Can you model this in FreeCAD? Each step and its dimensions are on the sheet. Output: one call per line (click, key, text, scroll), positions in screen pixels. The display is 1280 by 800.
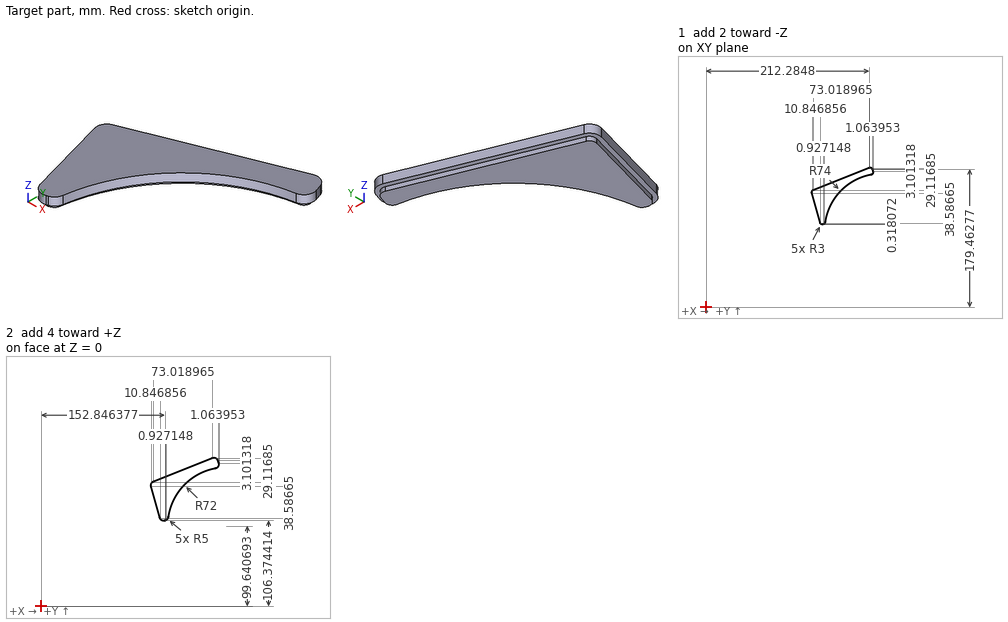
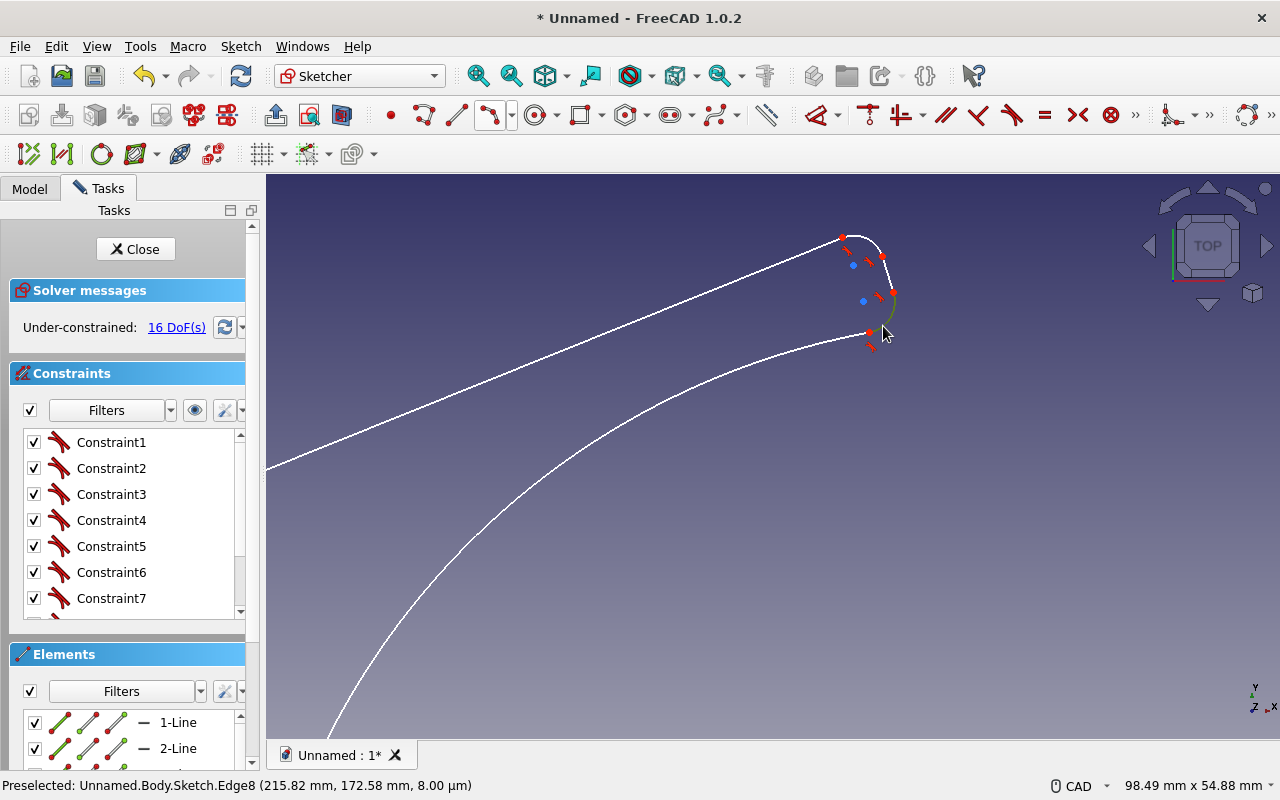
click(875, 244)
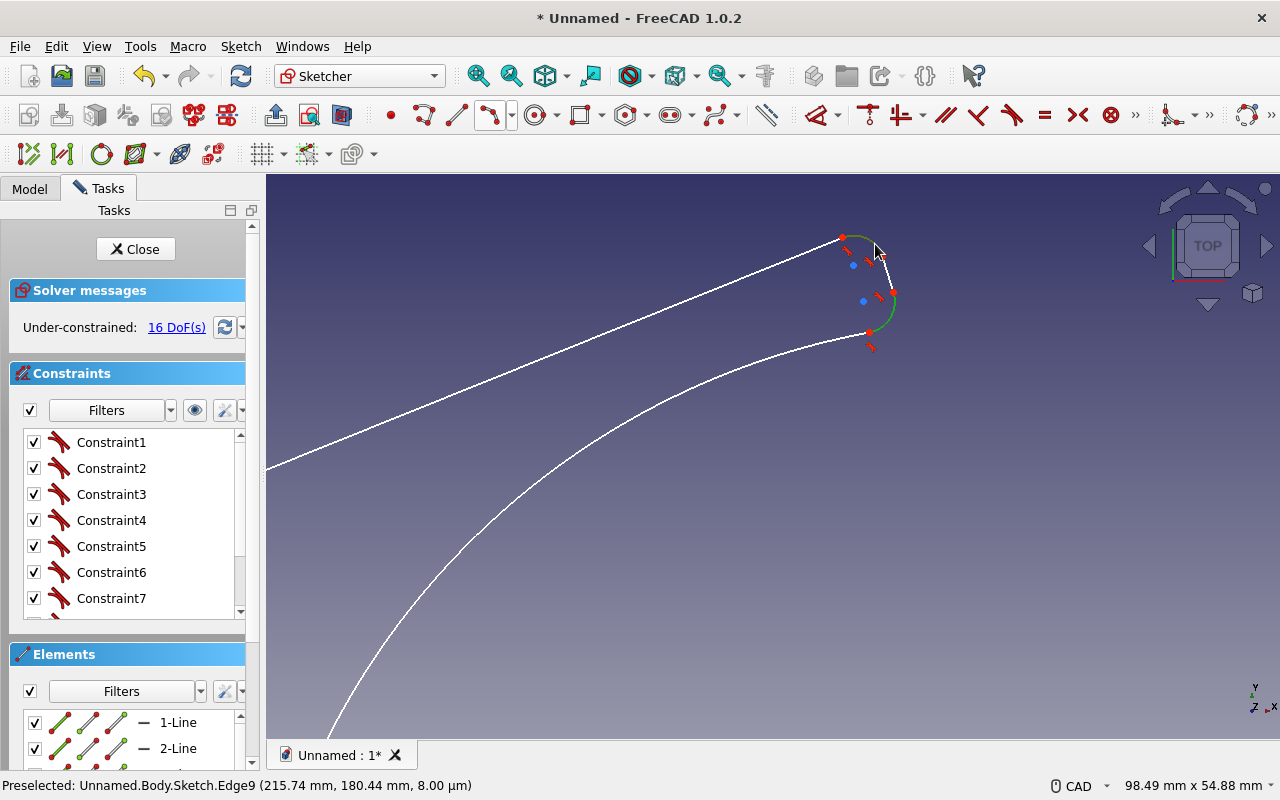
scroll(885, 326, down, 4)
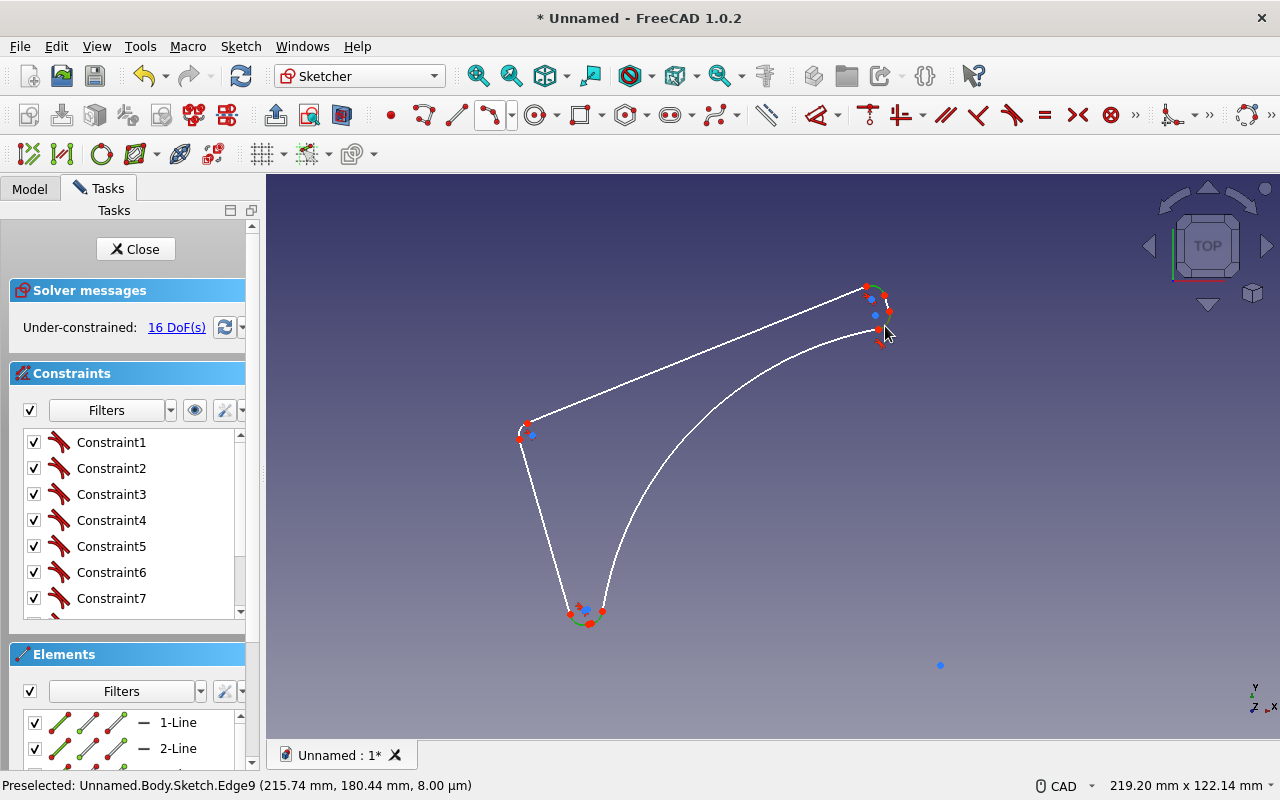
scroll(522, 426, up, 5)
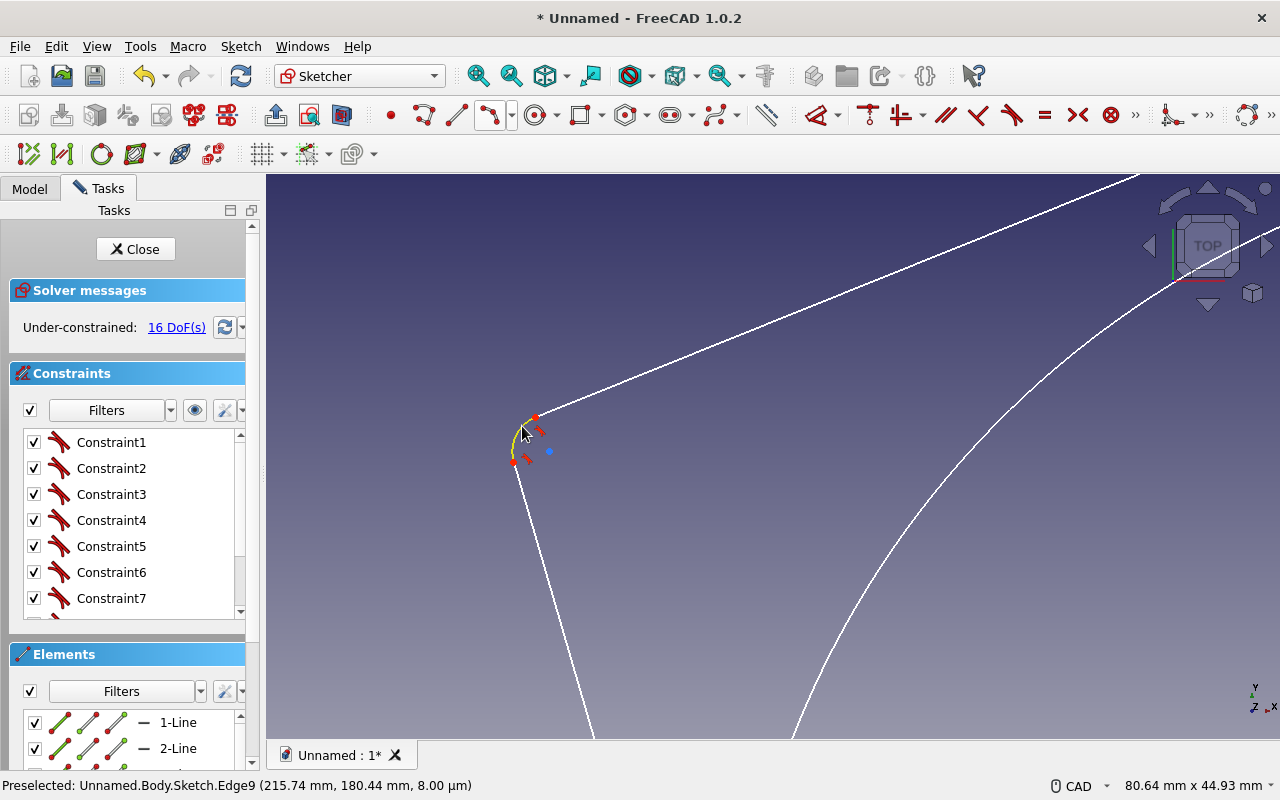
click(522, 426)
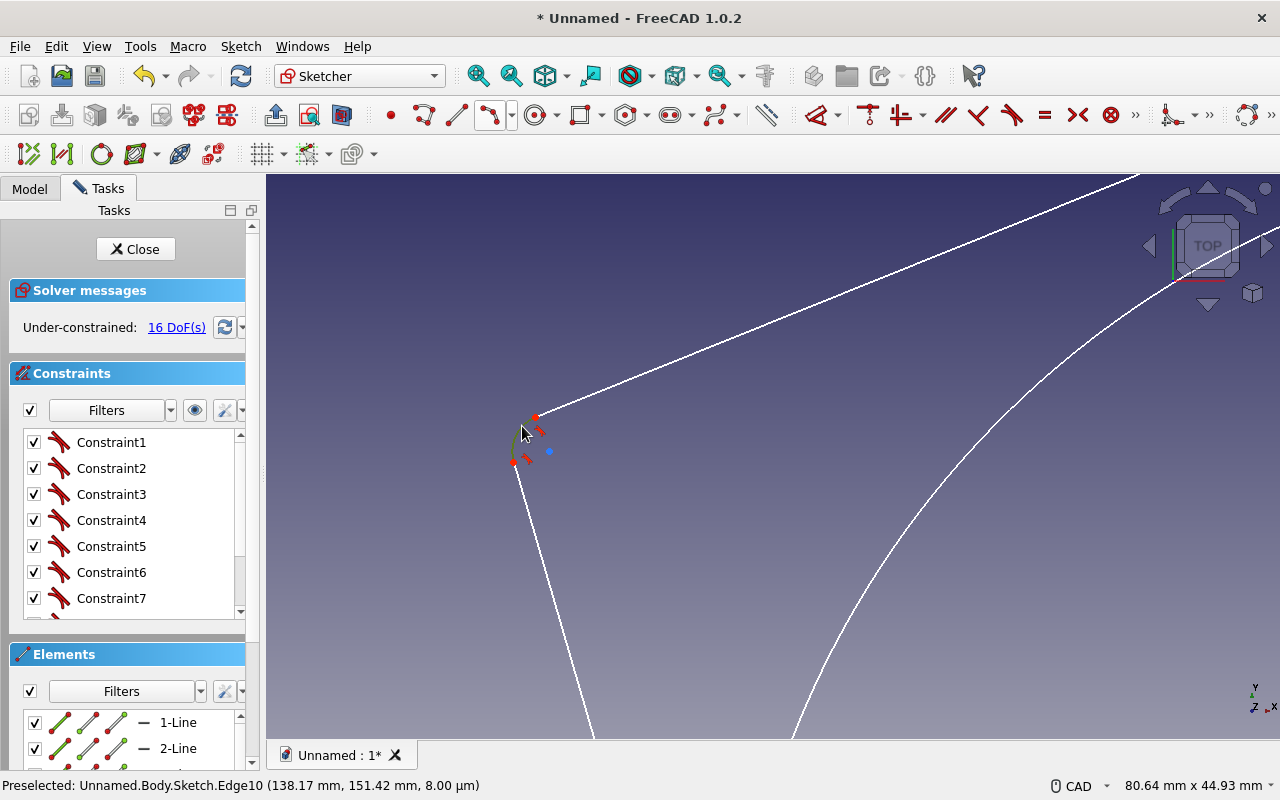
click(1045, 116)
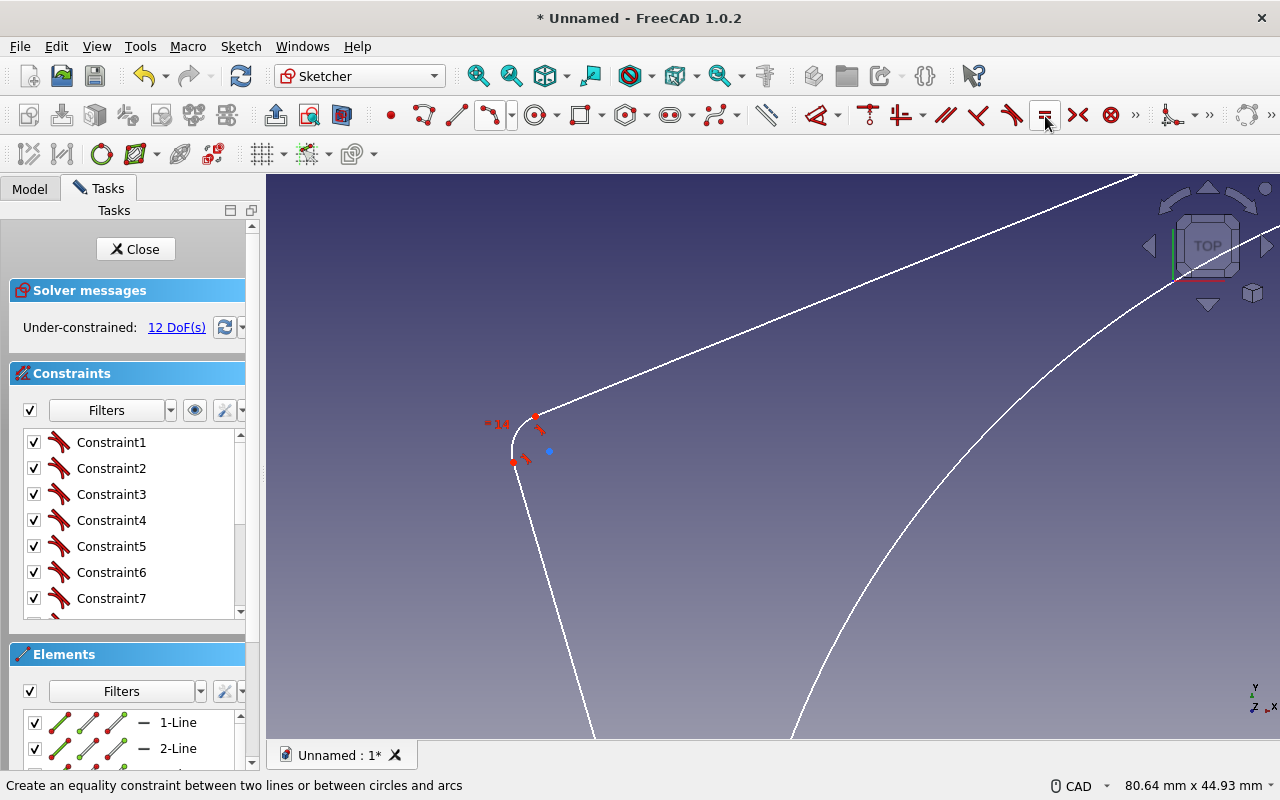
click(816, 116)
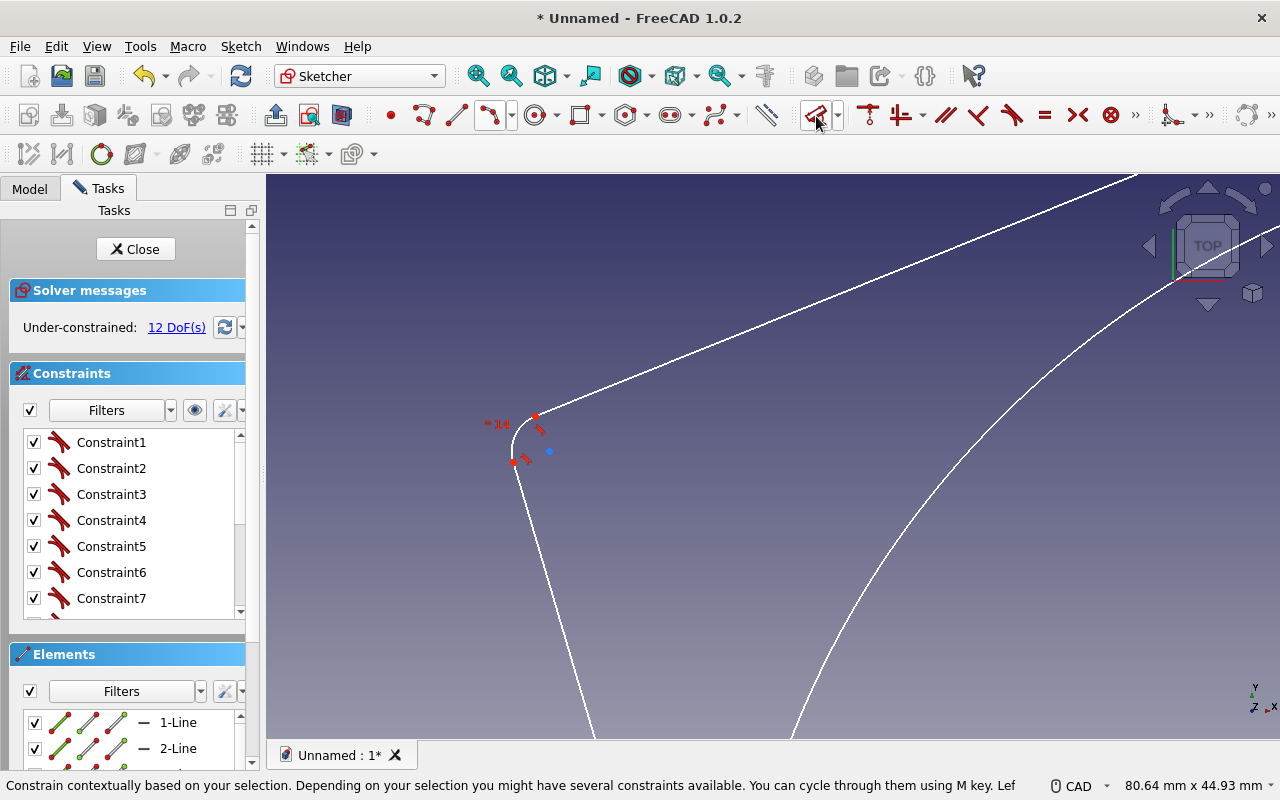
scroll(522, 426, down, 5)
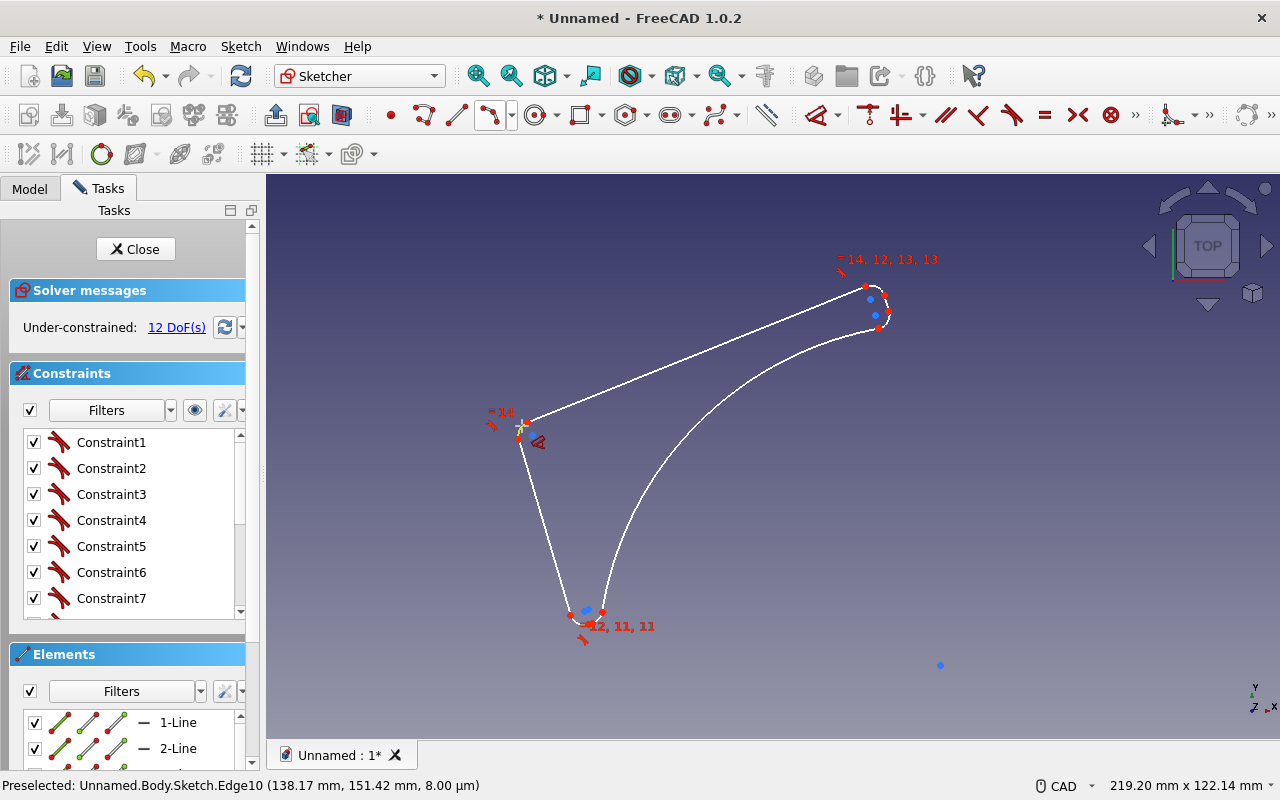
scroll(574, 621, up, 6)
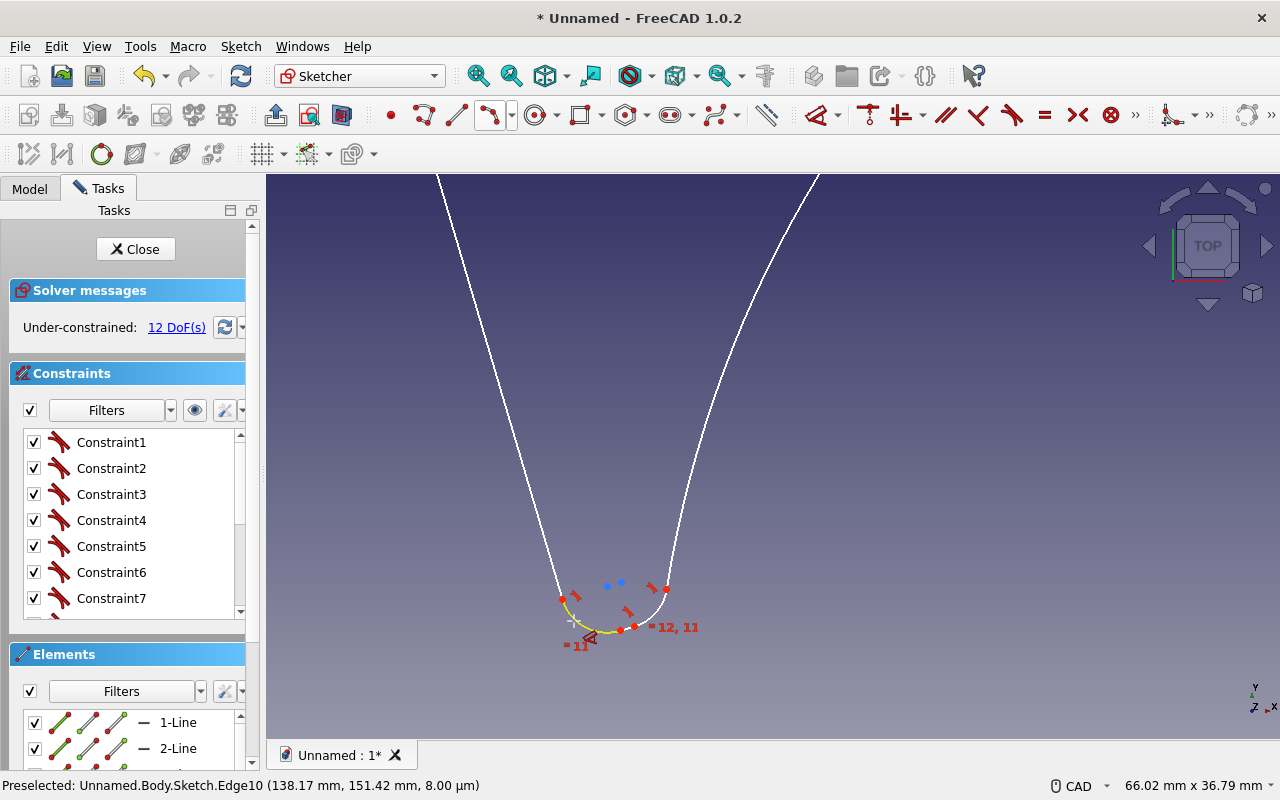
click(573, 618)
click(550, 640)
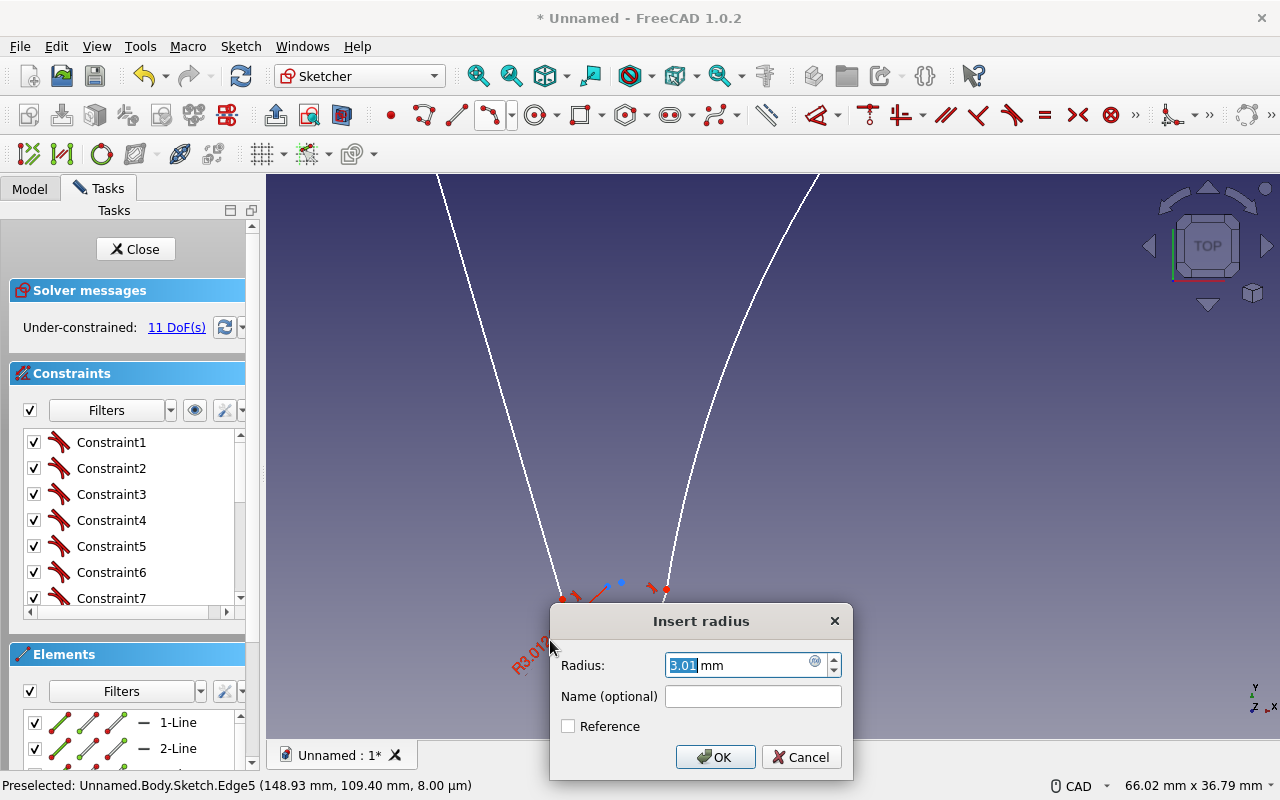
text(3)
key(Return)